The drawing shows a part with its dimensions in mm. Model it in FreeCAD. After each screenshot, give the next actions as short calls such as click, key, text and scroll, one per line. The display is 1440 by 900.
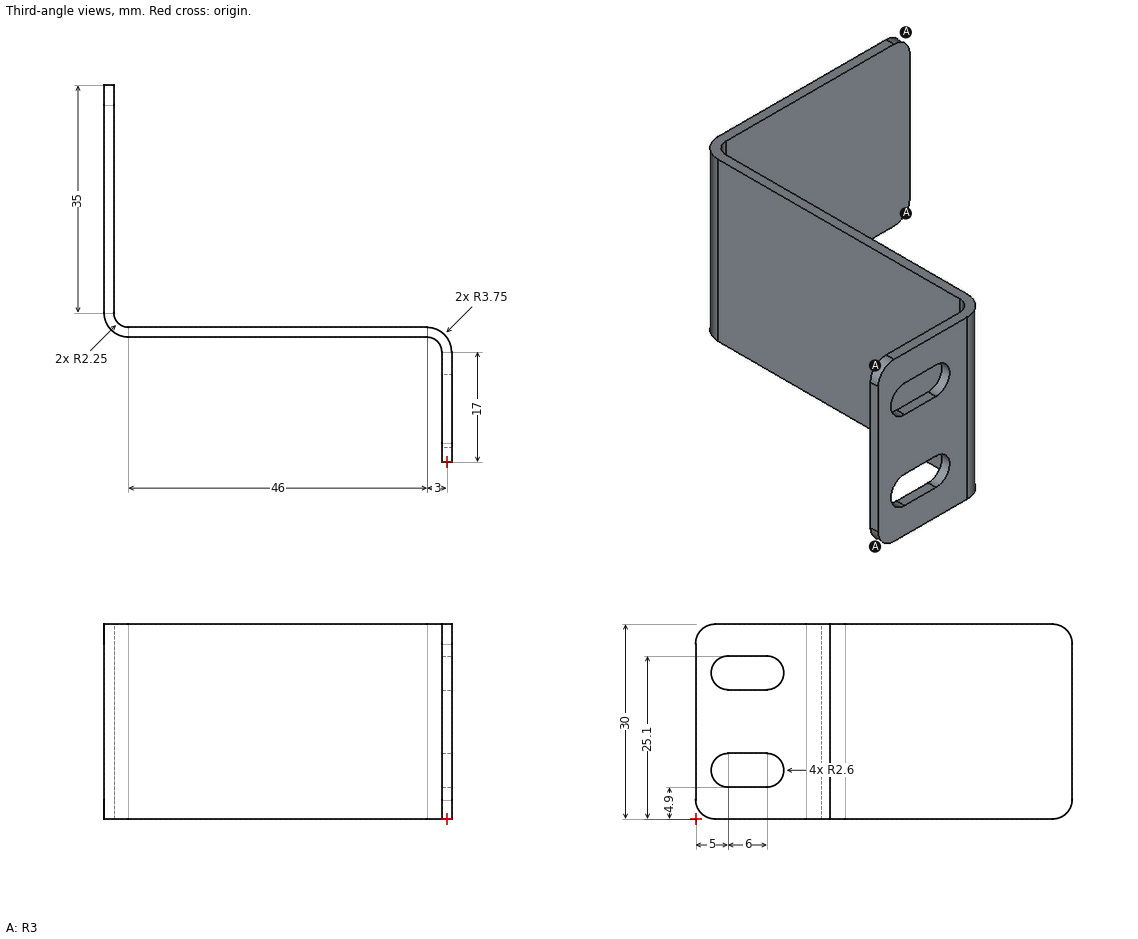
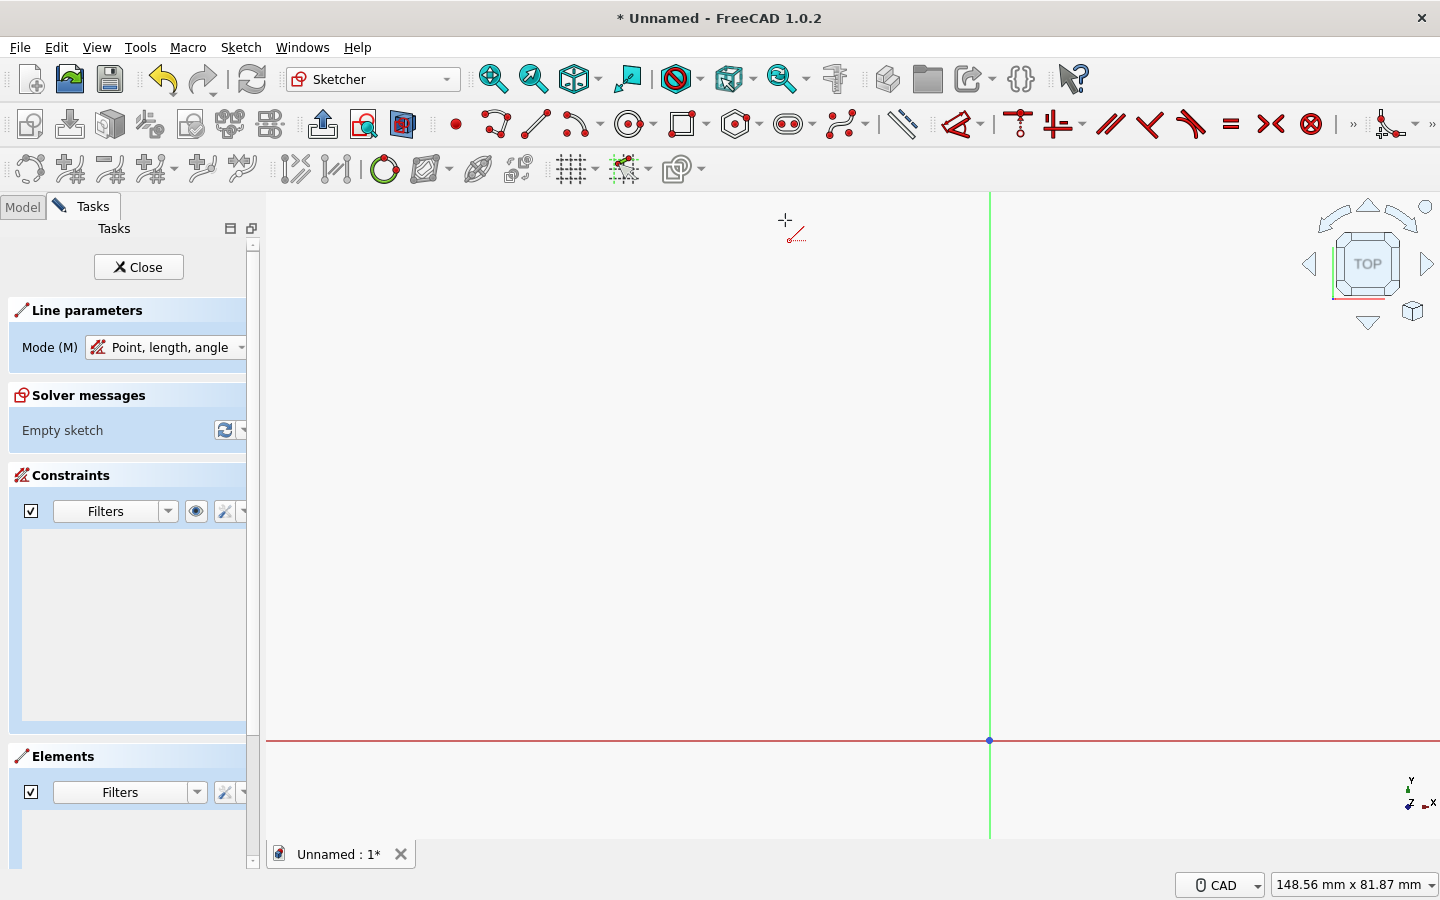
click(966, 577)
click(603, 577)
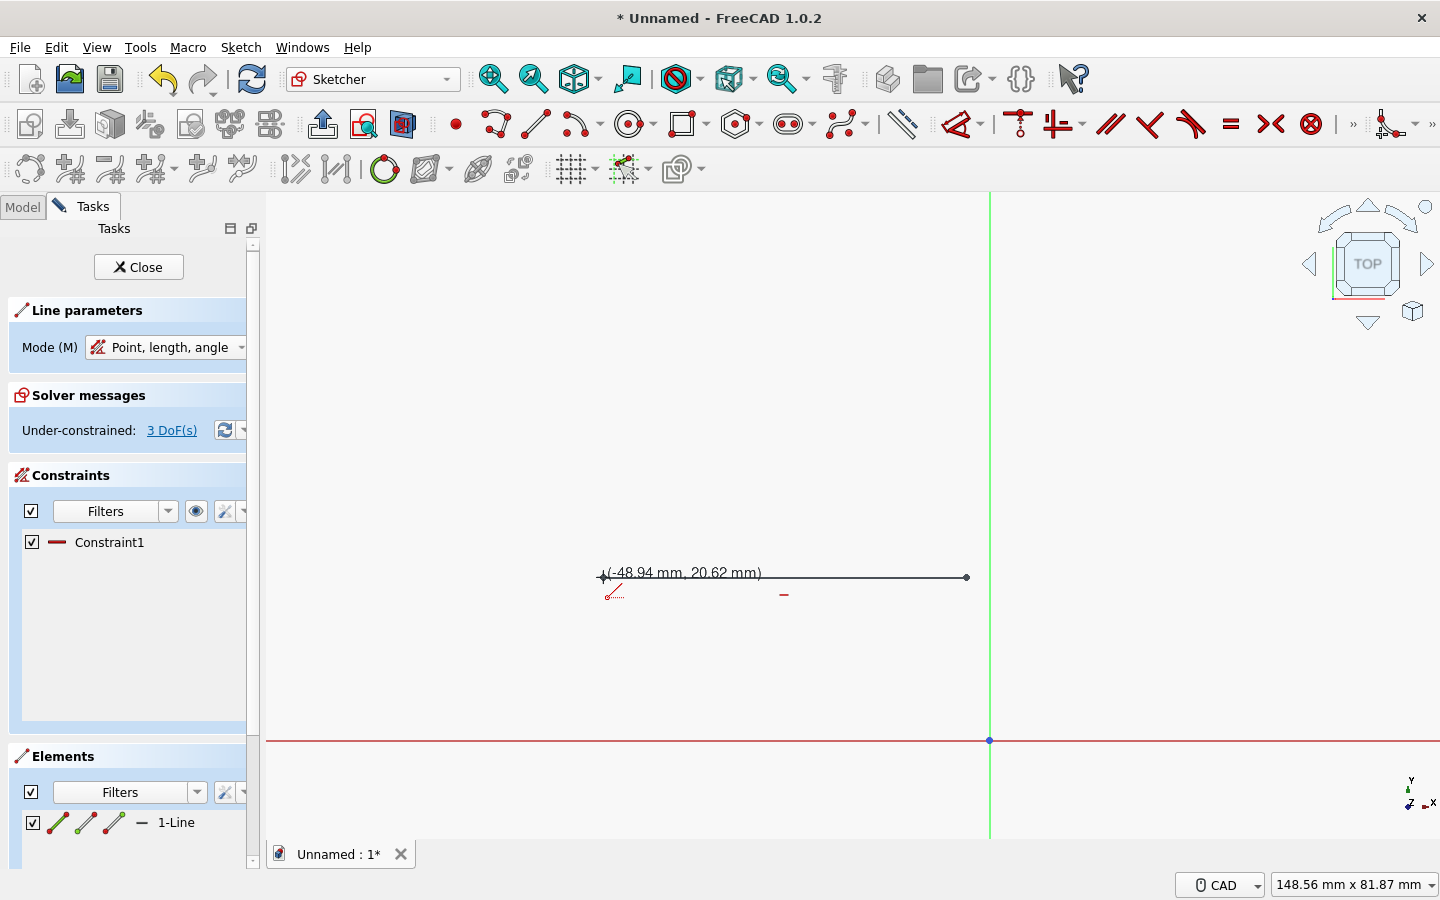
click(496, 124)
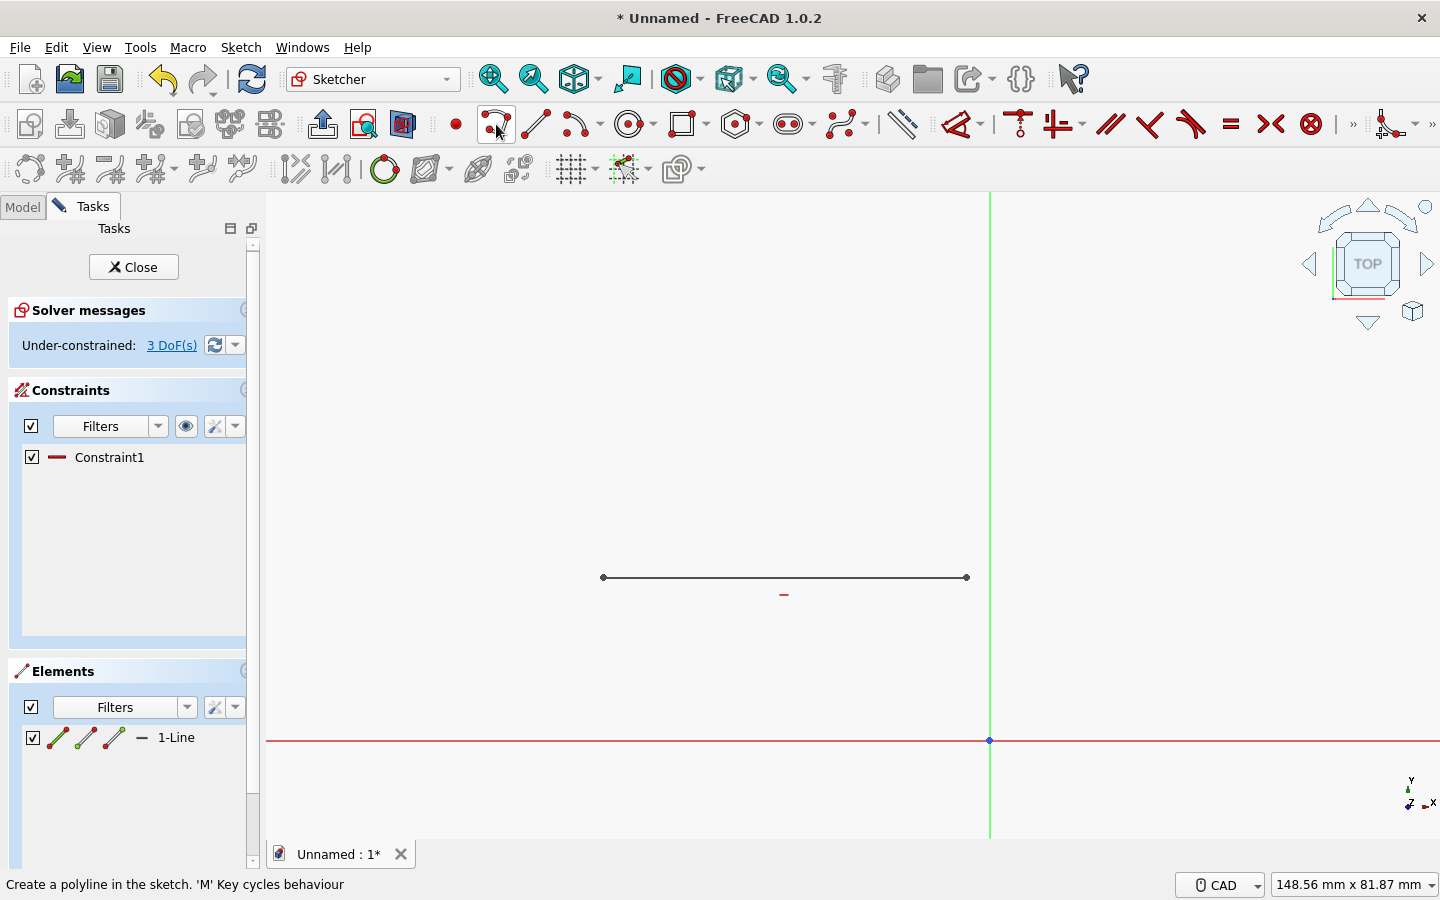
click(585, 559)
click(585, 283)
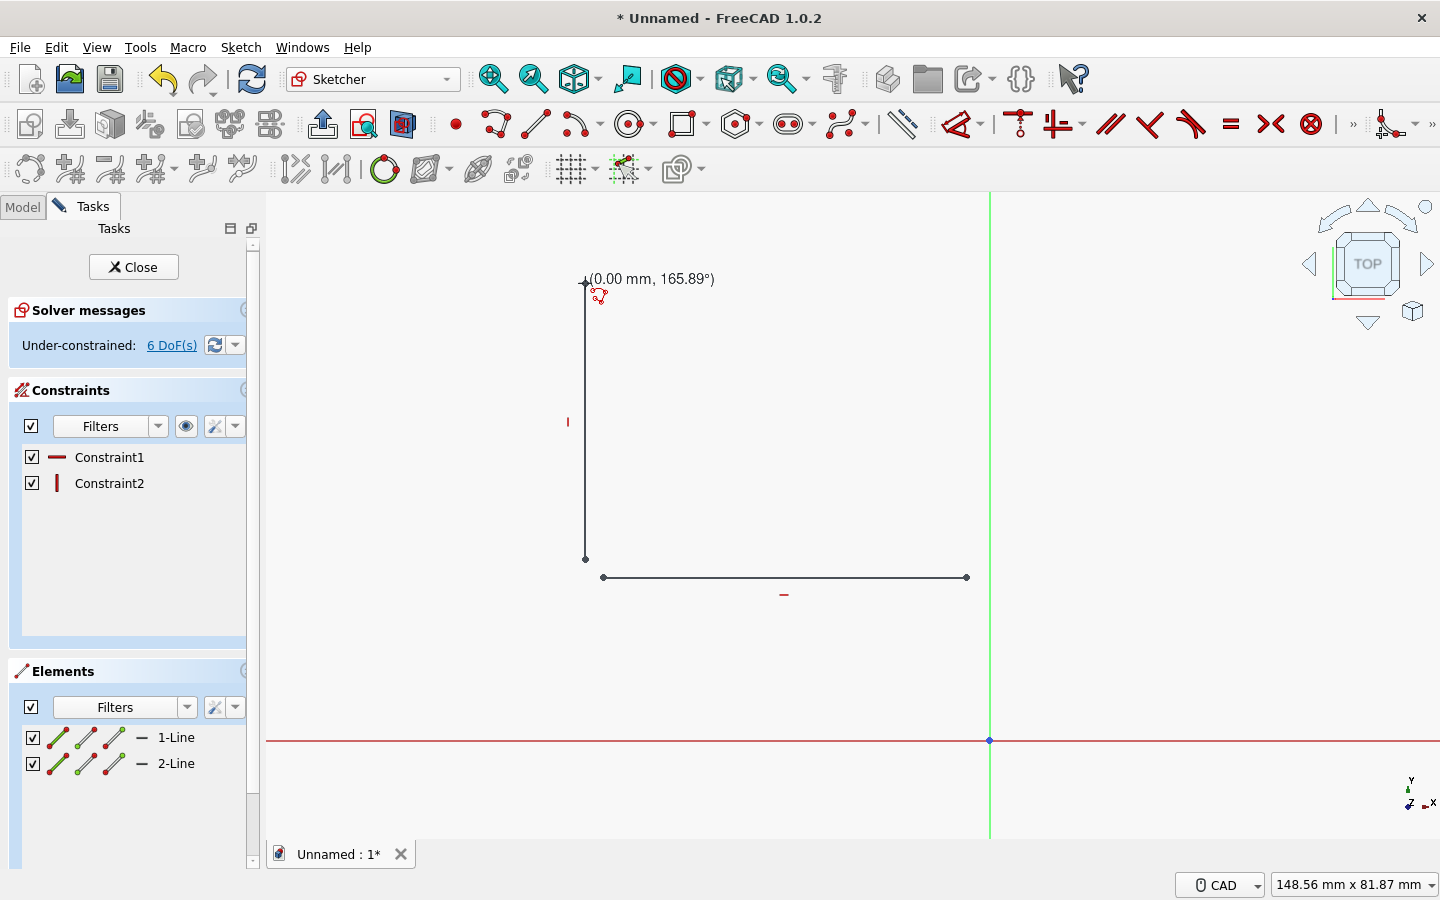
scroll(573, 283, up, 2)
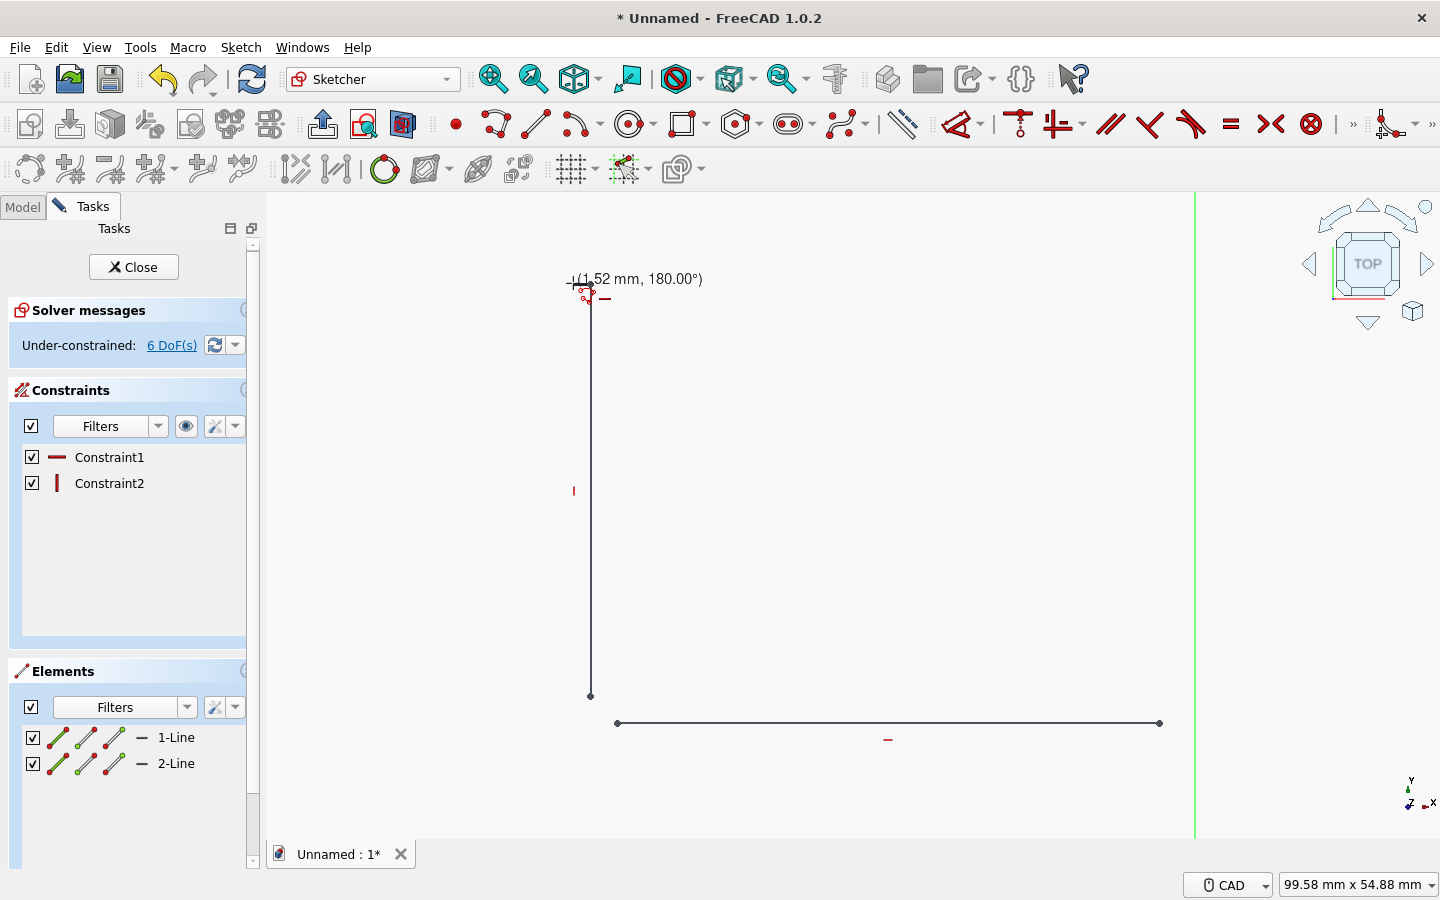
click(573, 283)
click(573, 695)
right_click(573, 695)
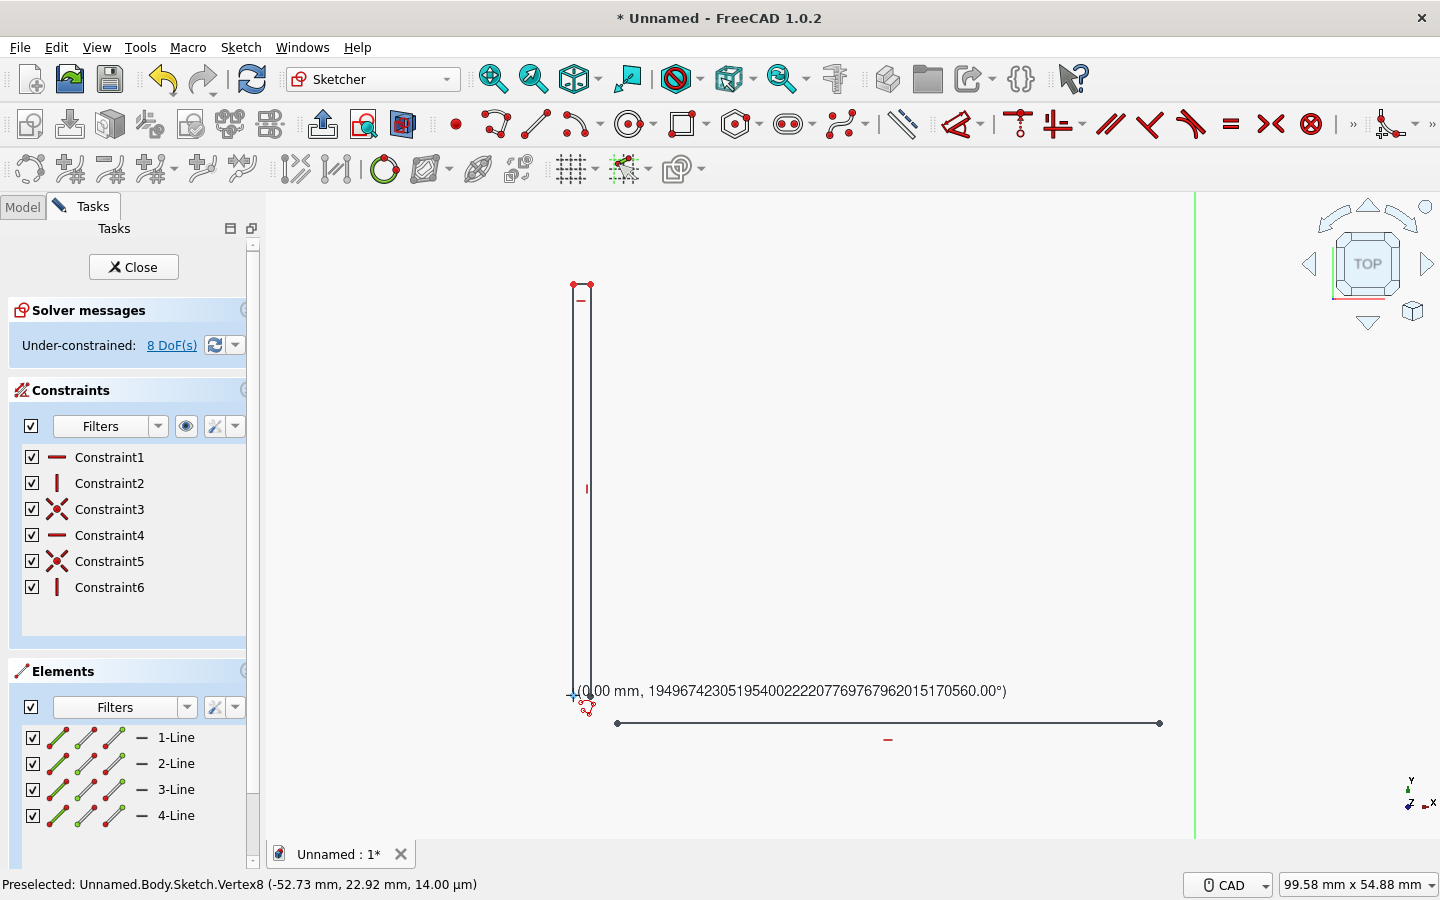
click(536, 124)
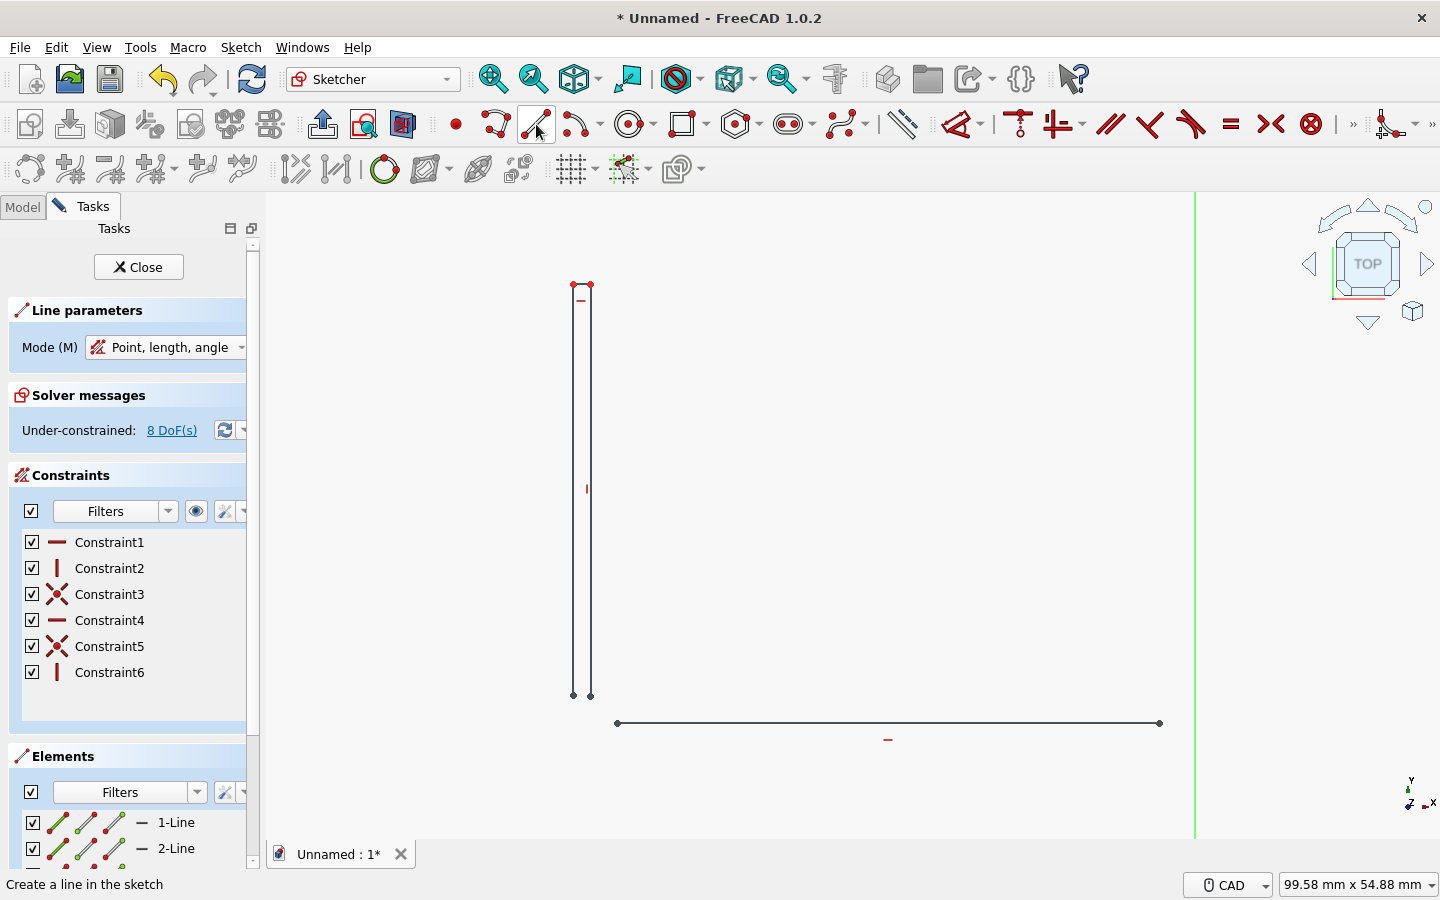
click(617, 739)
click(1159, 739)